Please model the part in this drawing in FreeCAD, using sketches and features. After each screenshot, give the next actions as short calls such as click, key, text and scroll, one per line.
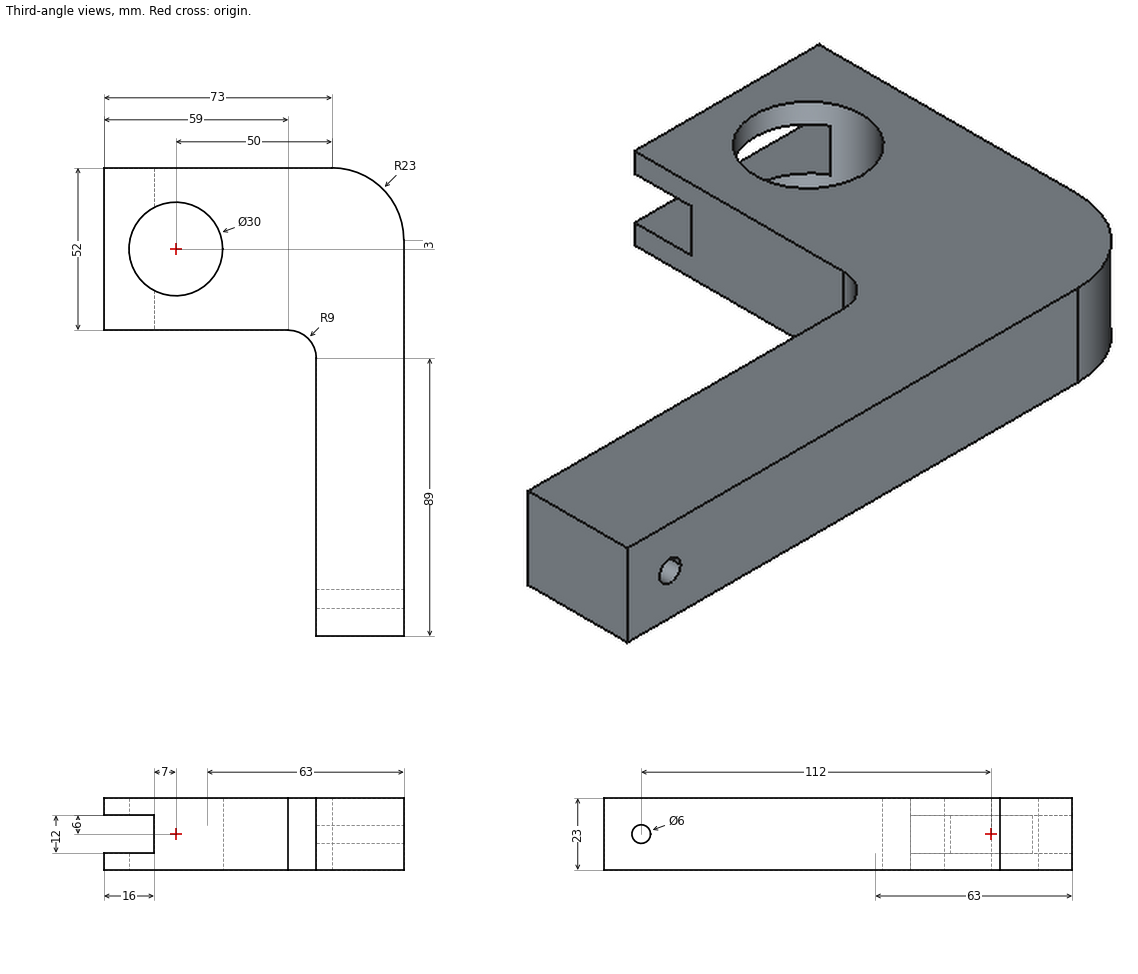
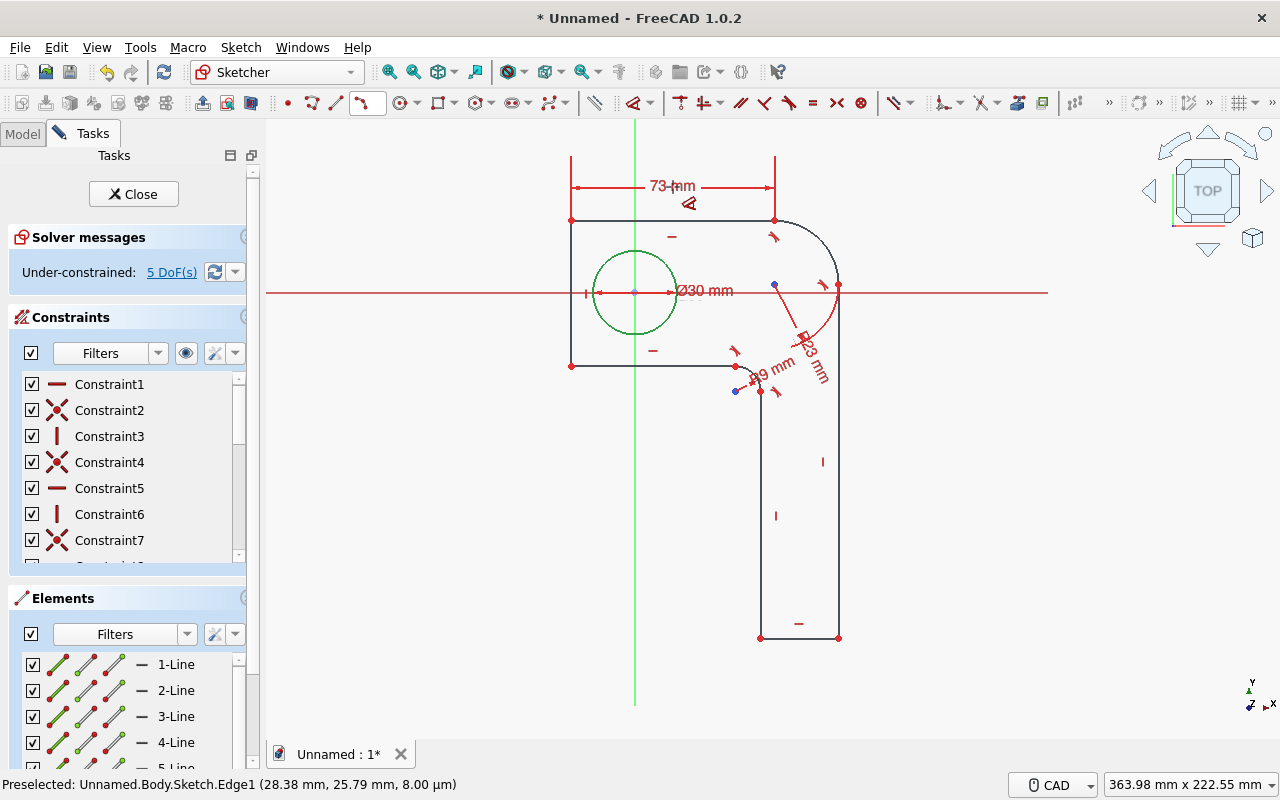
click(571, 264)
click(537, 260)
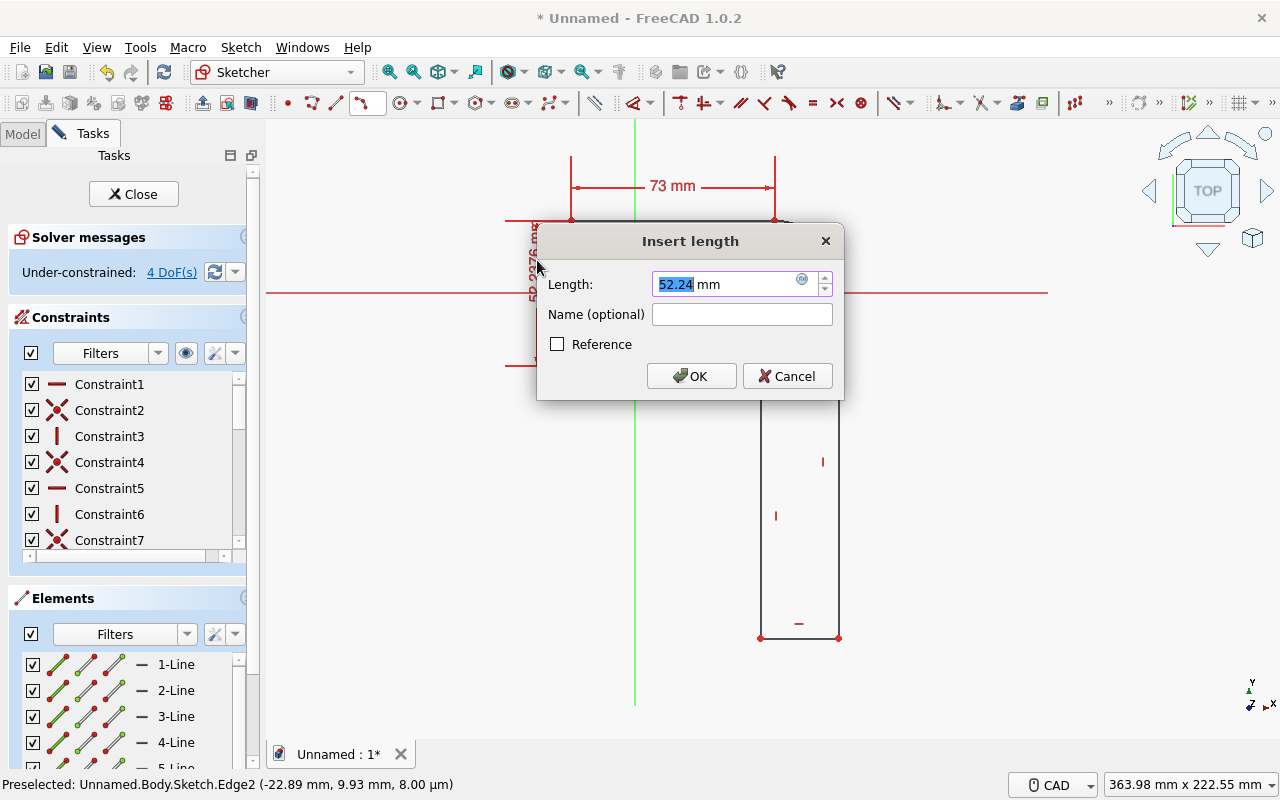
text(52)
key(Return)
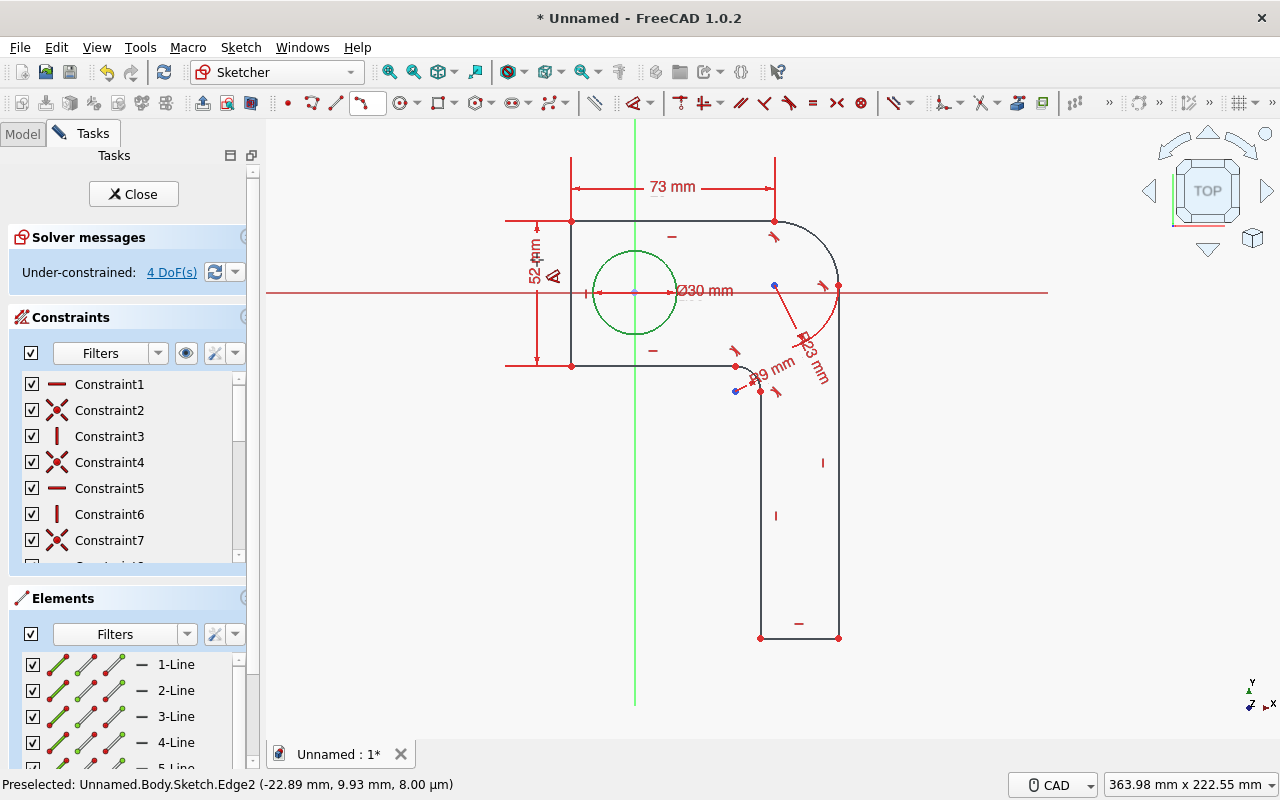
click(620, 366)
click(691, 332)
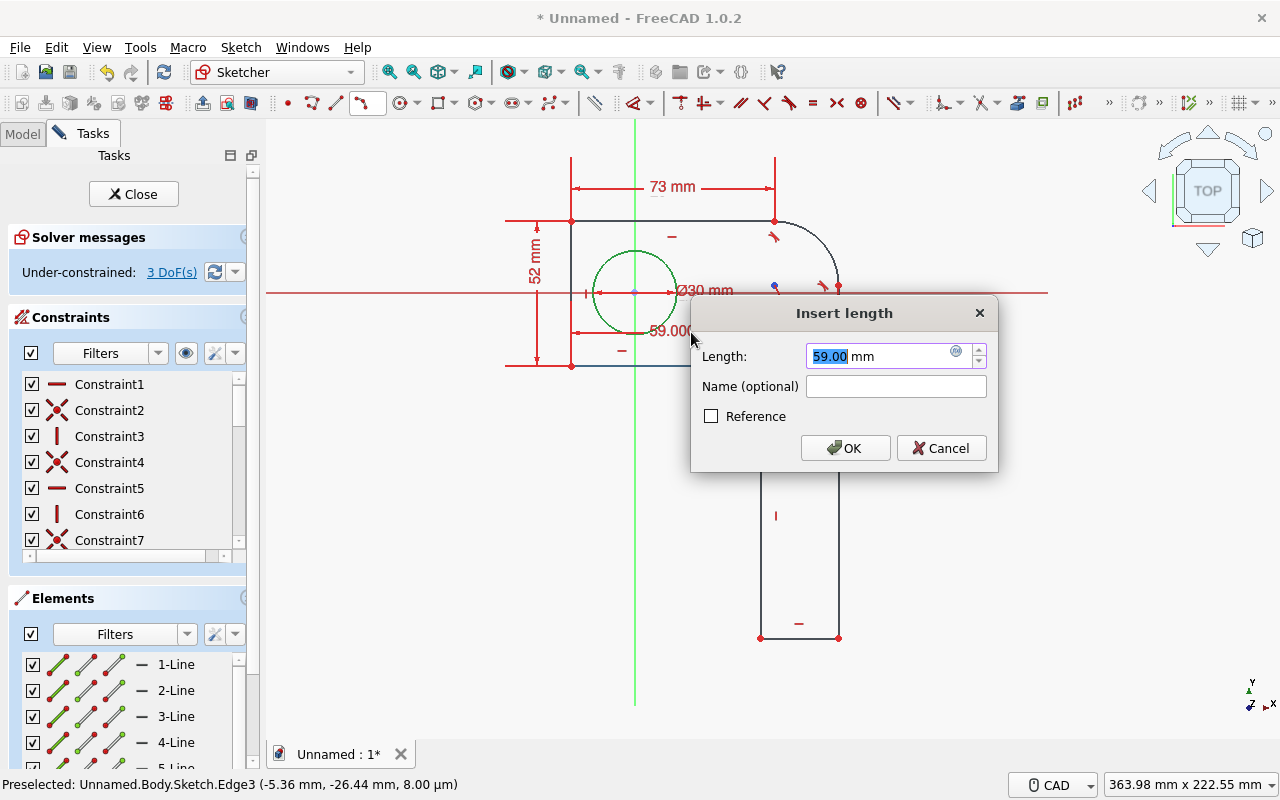
text(59)
key(Return)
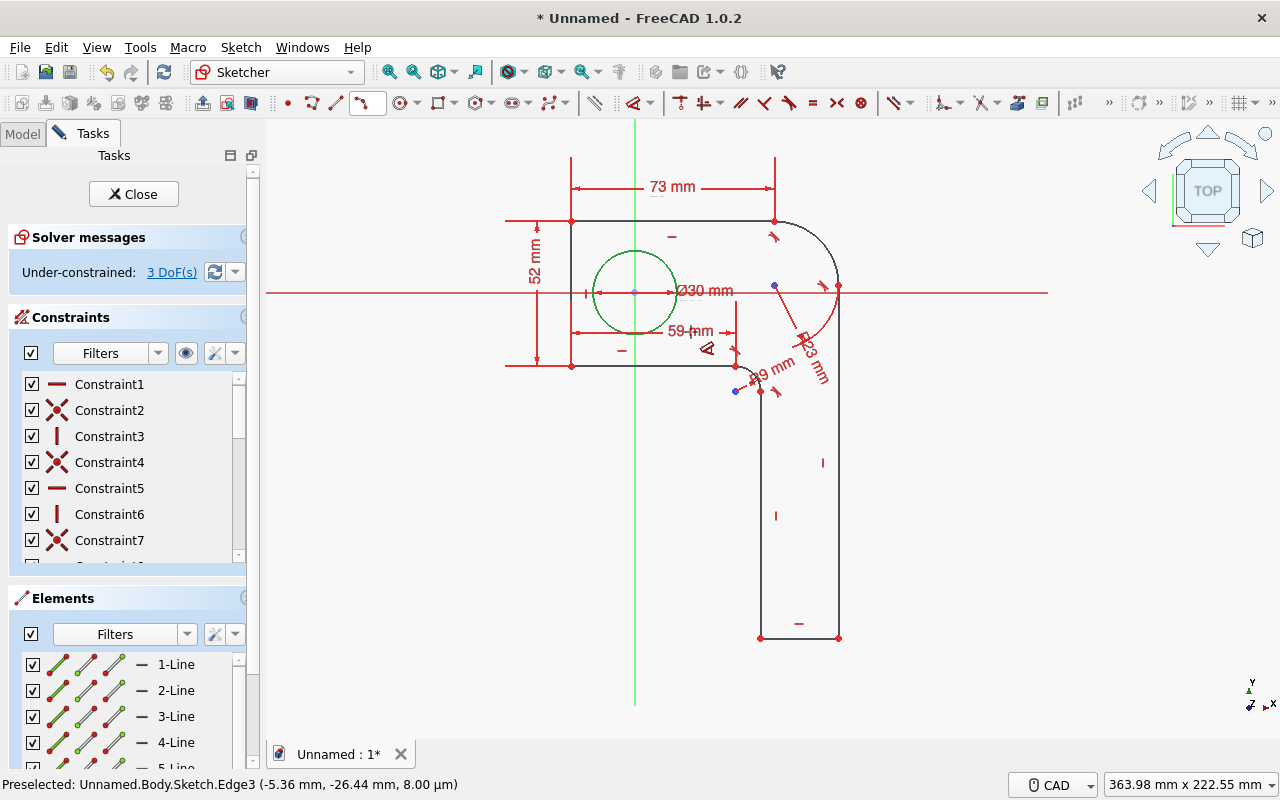
click(761, 466)
click(795, 515)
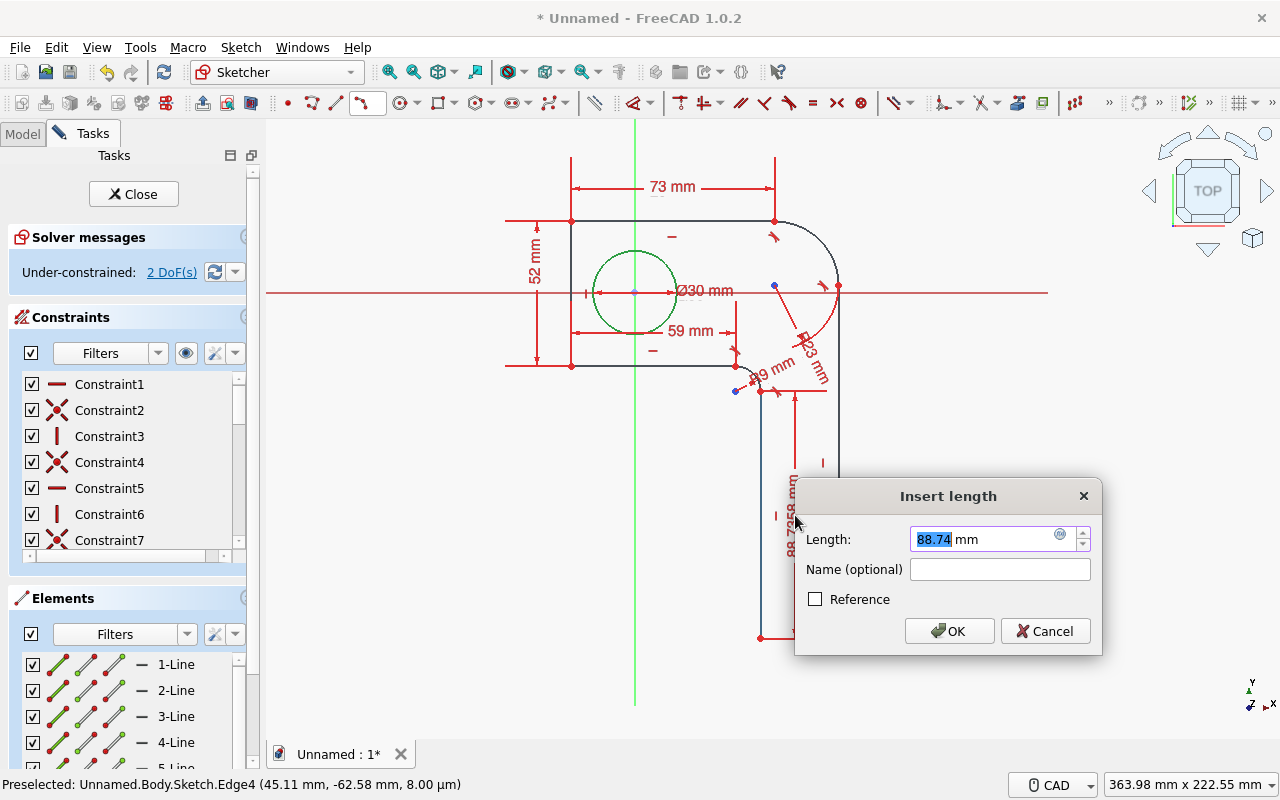
text(89)
key(Return)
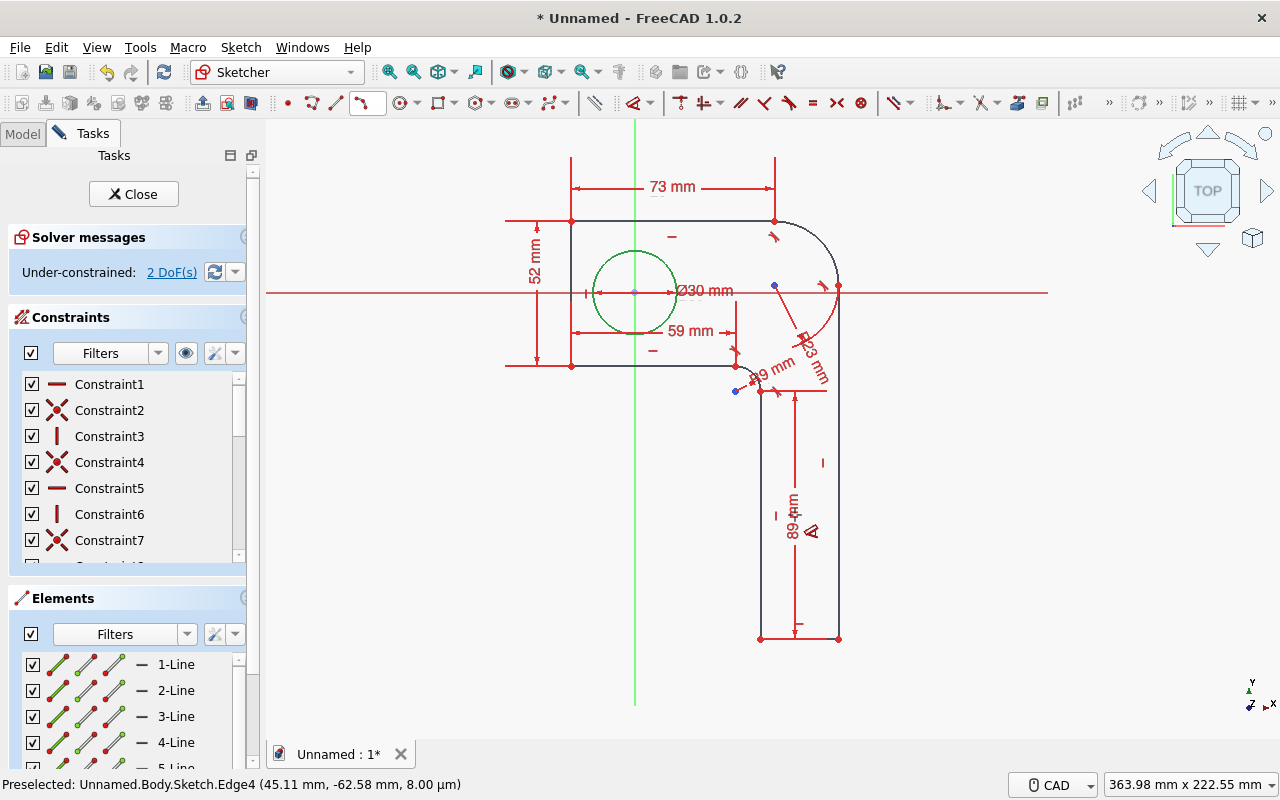
scroll(839, 286, up, 8)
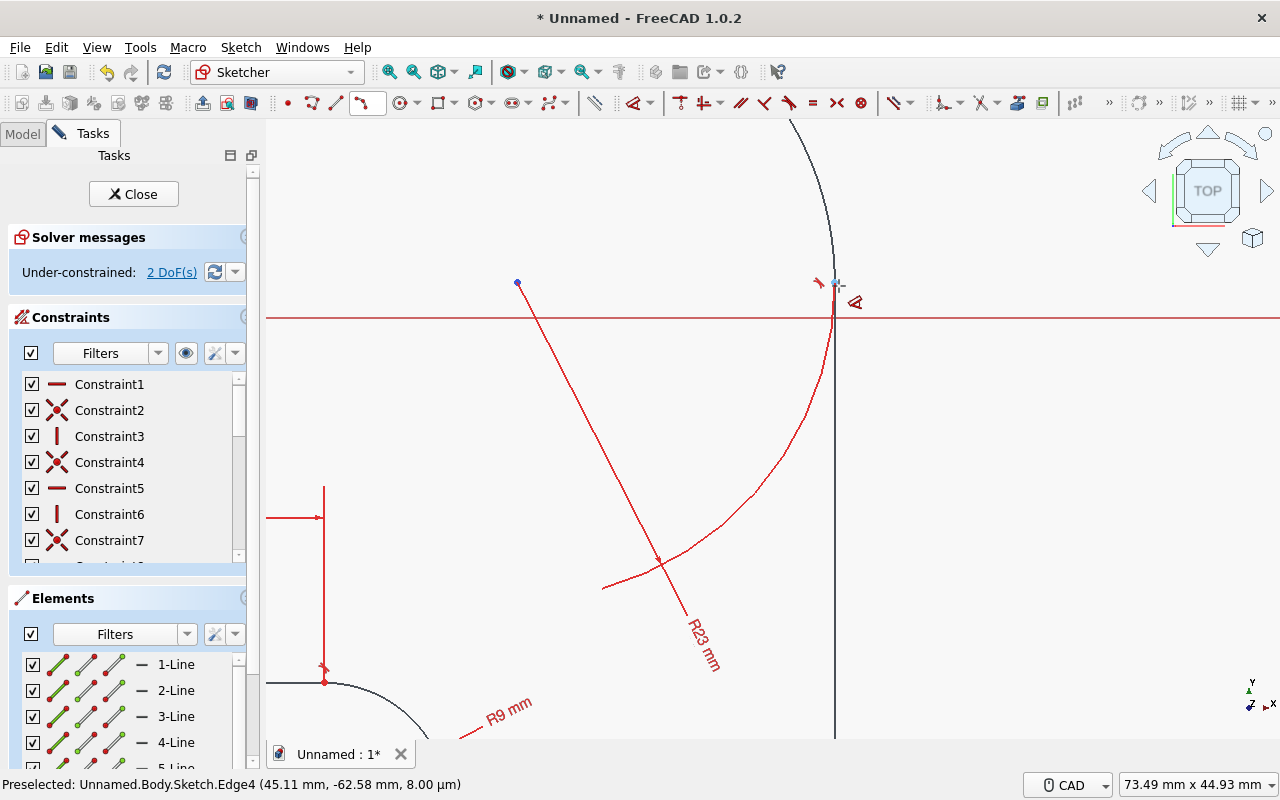
click(835, 283)
click(869, 300)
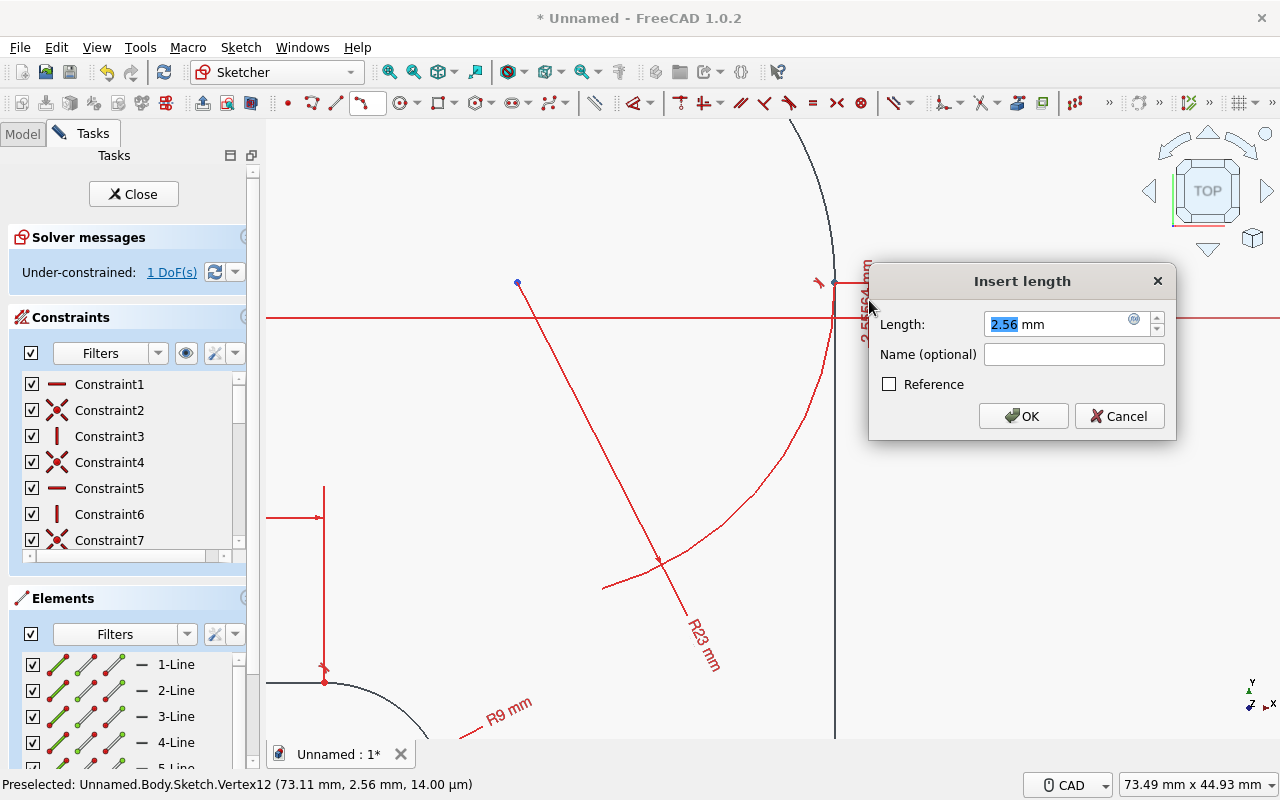
text(3)
key(Return)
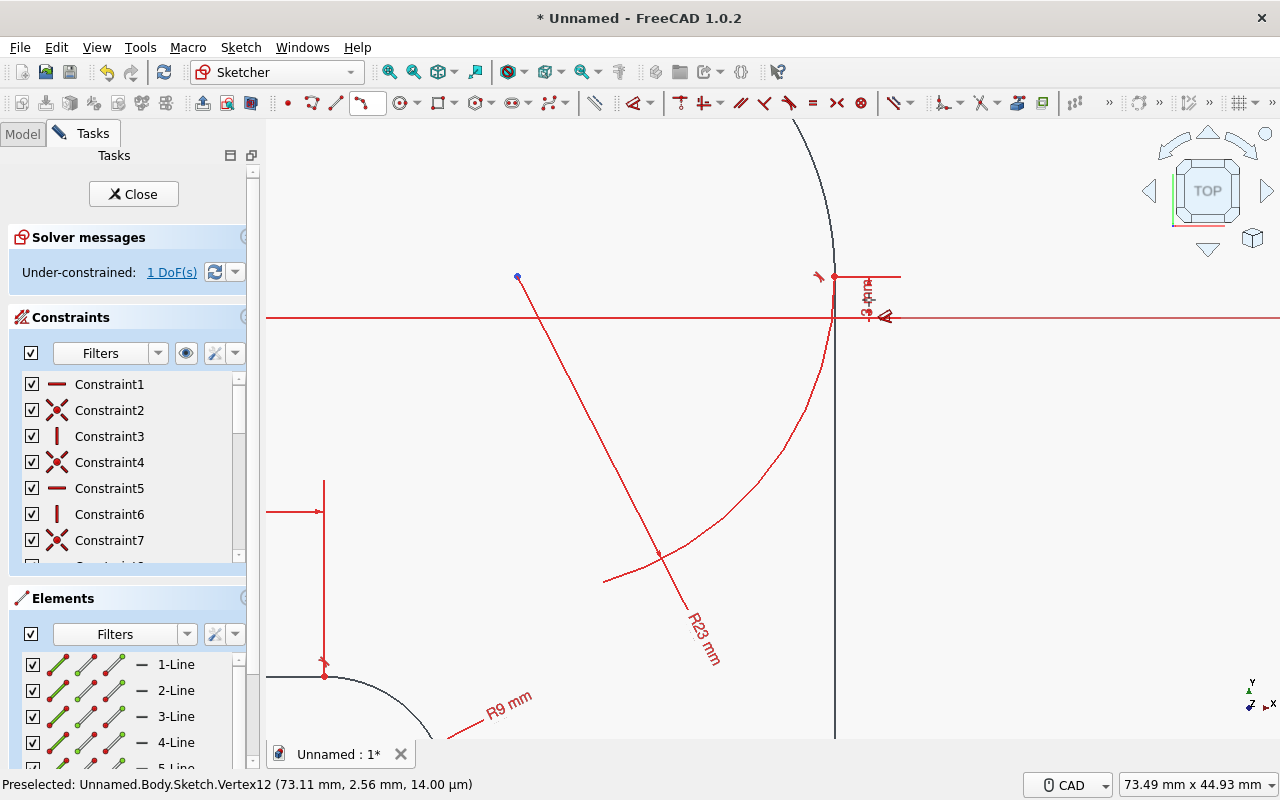
scroll(839, 286, down, 8)